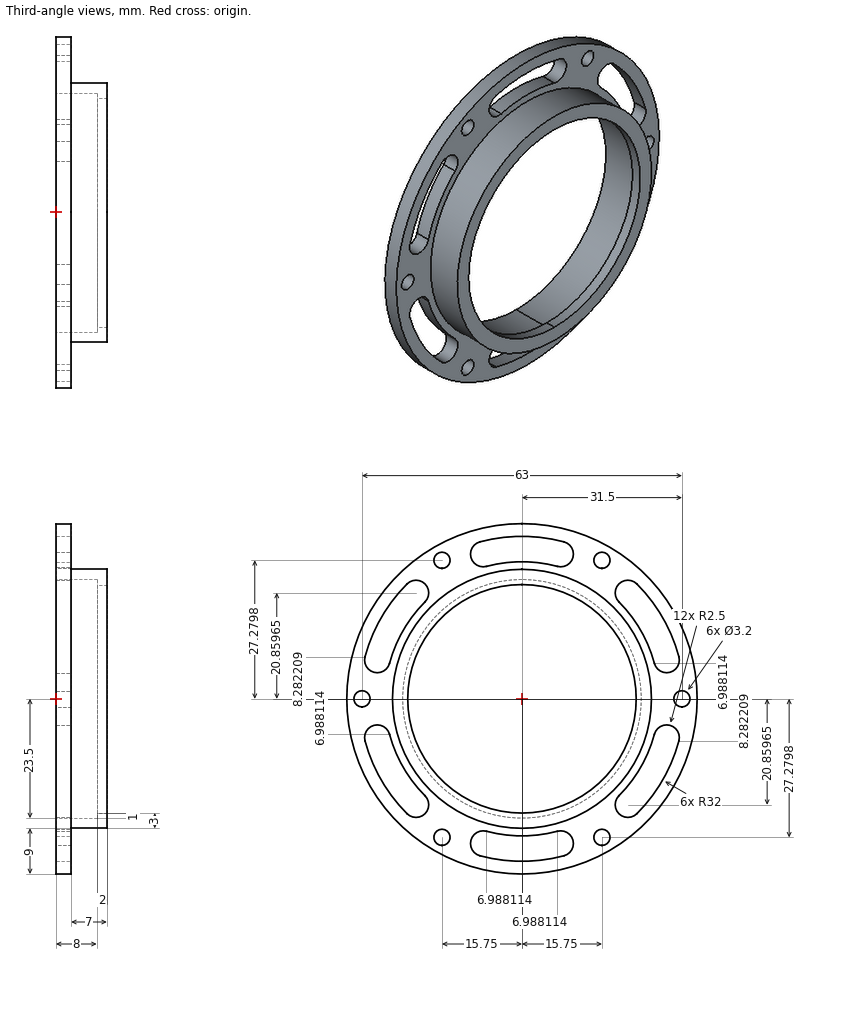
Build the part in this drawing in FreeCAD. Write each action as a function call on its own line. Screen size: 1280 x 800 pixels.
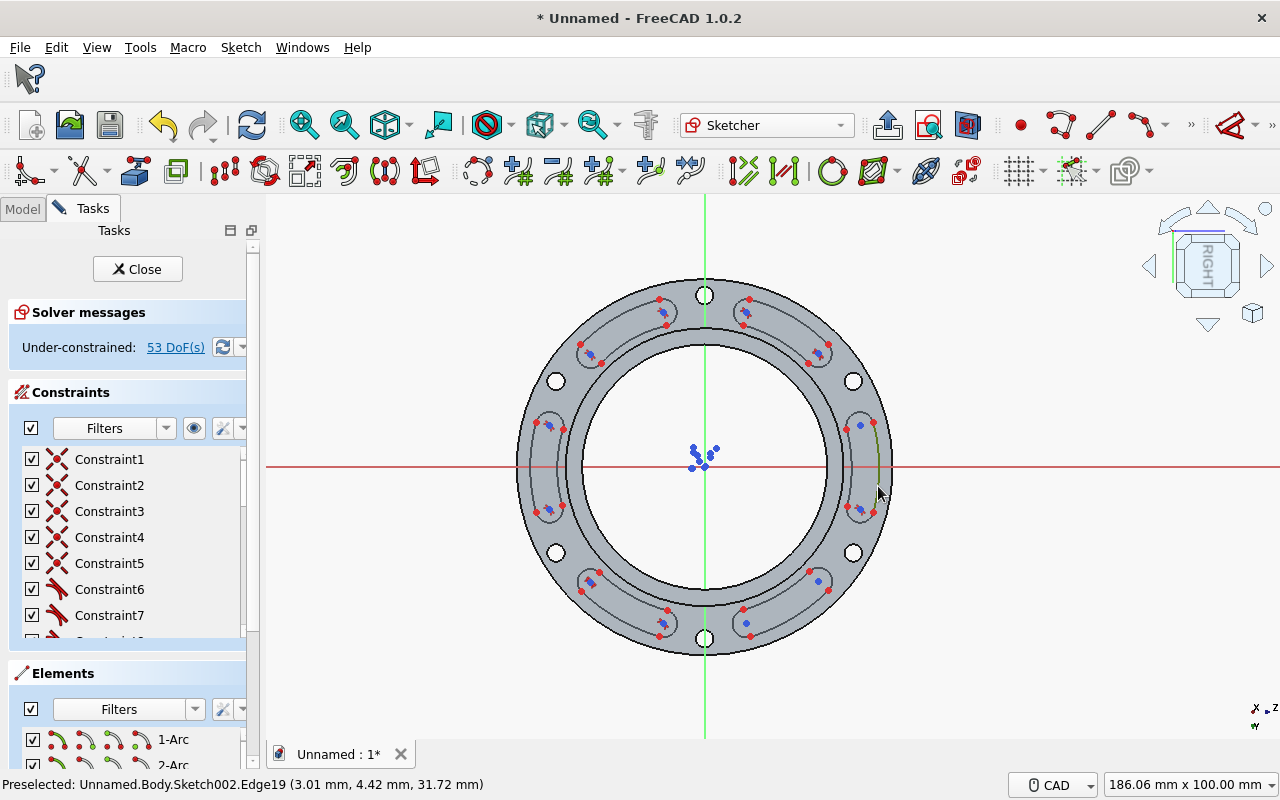
click(865, 413)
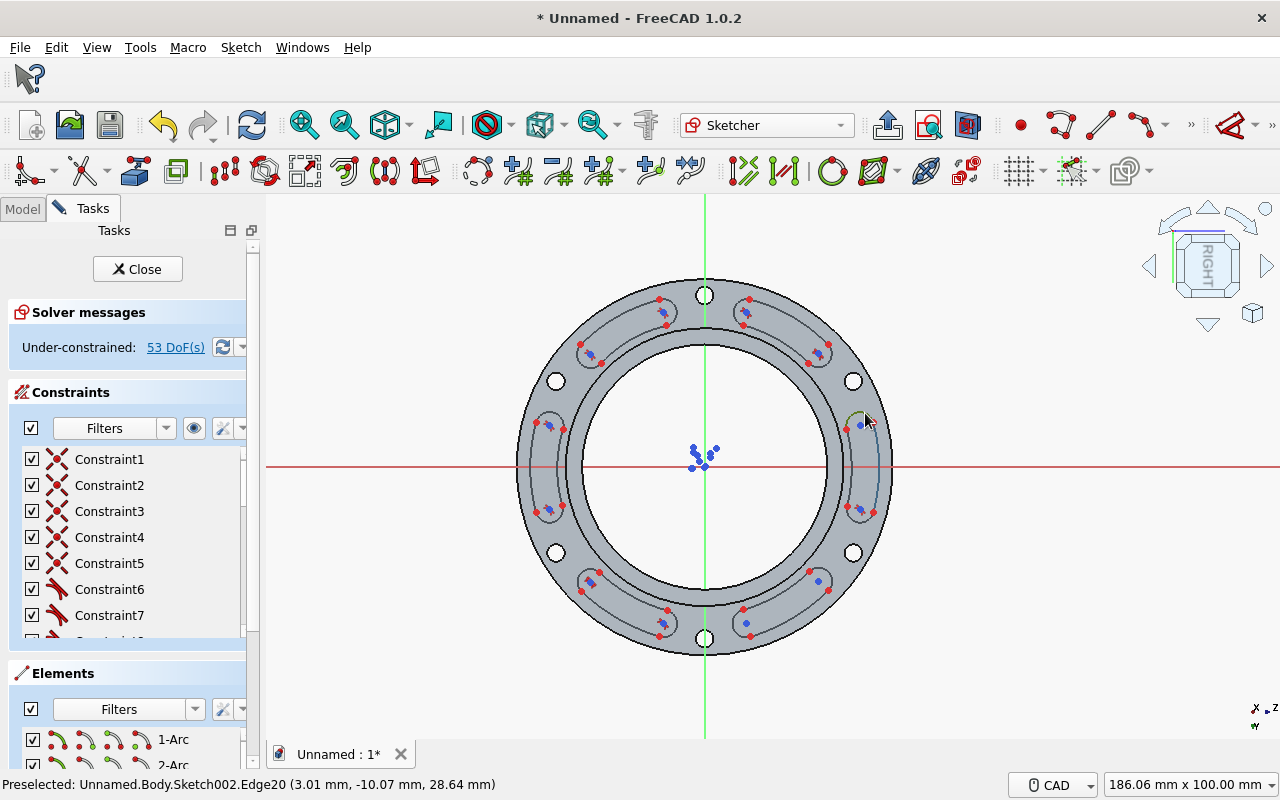
key(t)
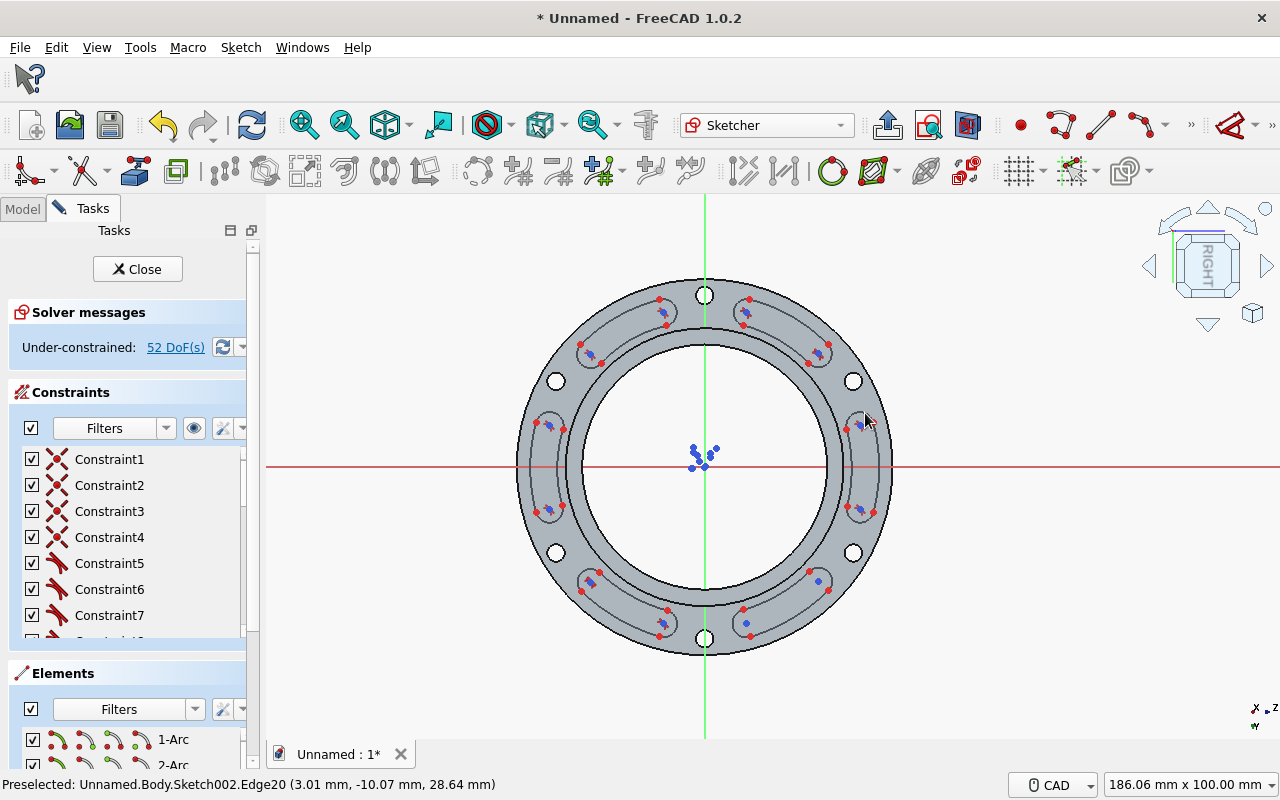
click(765, 602)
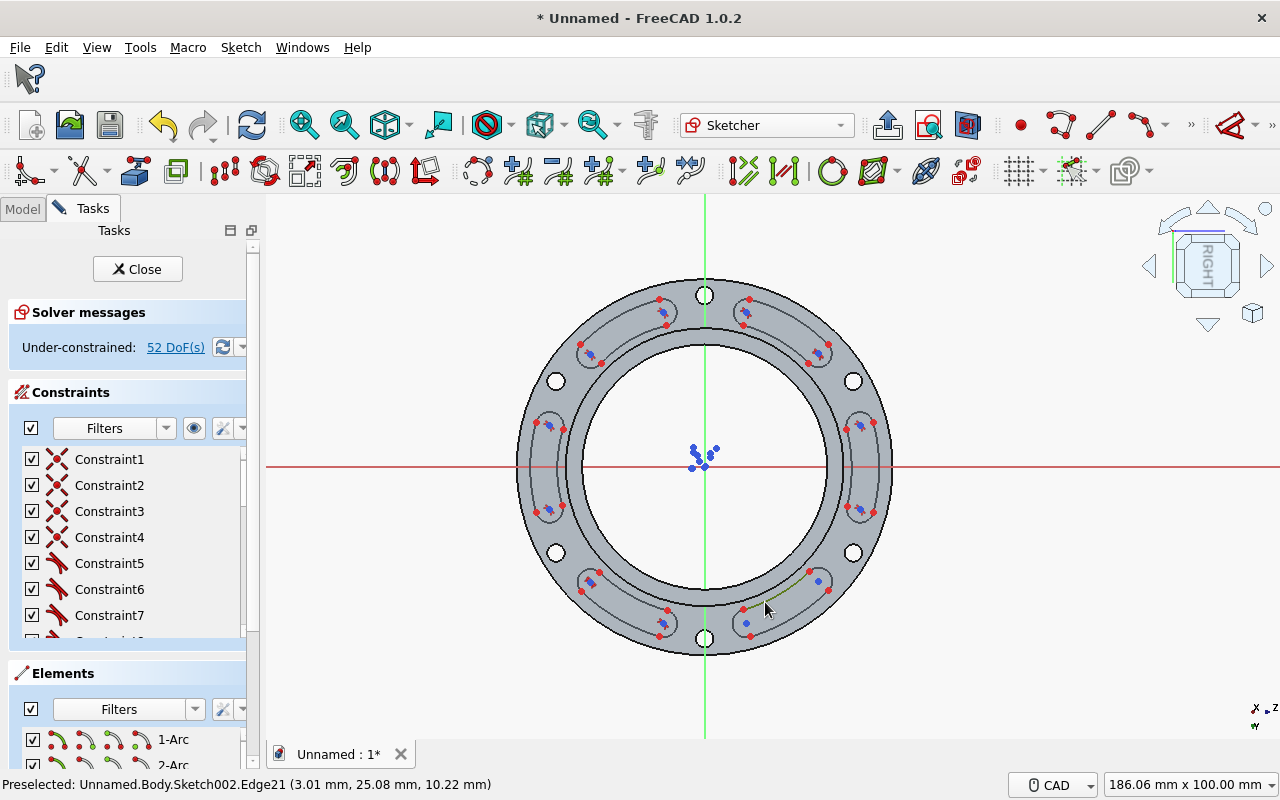
click(734, 618)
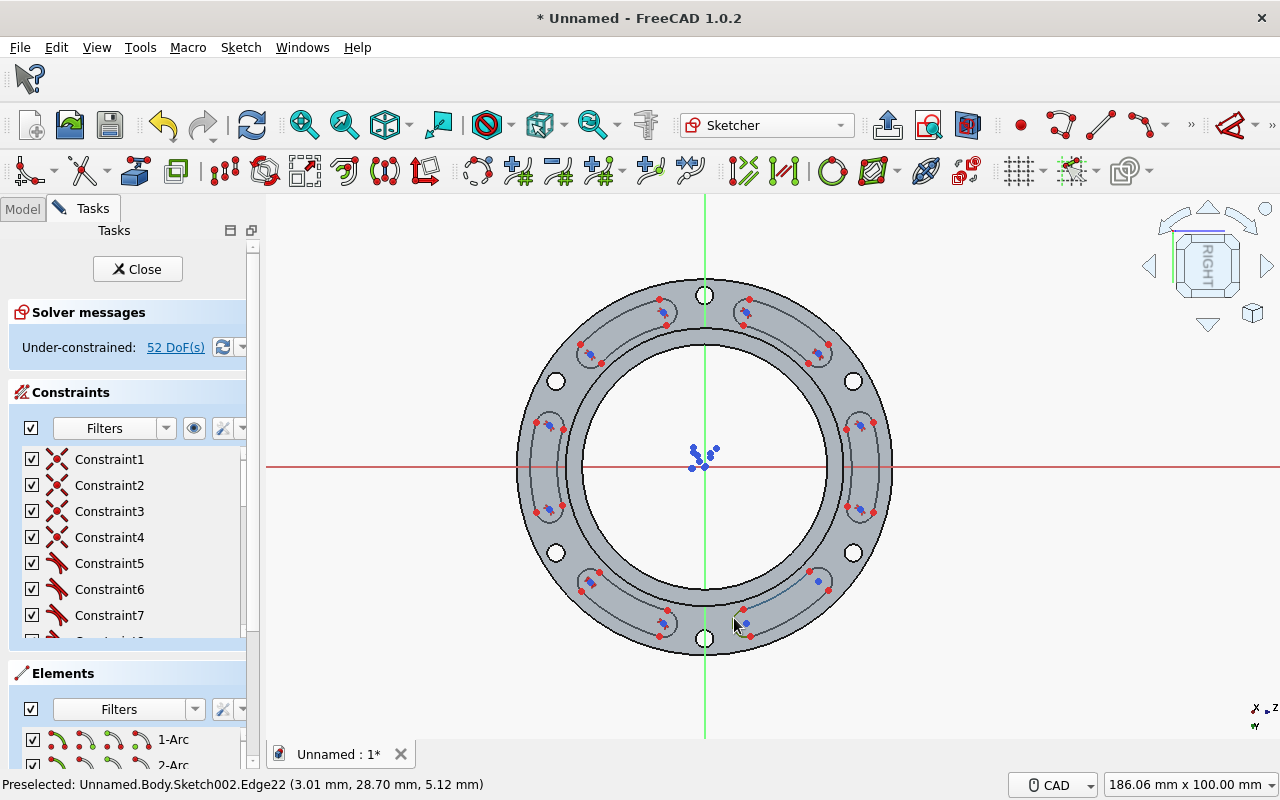
key(t)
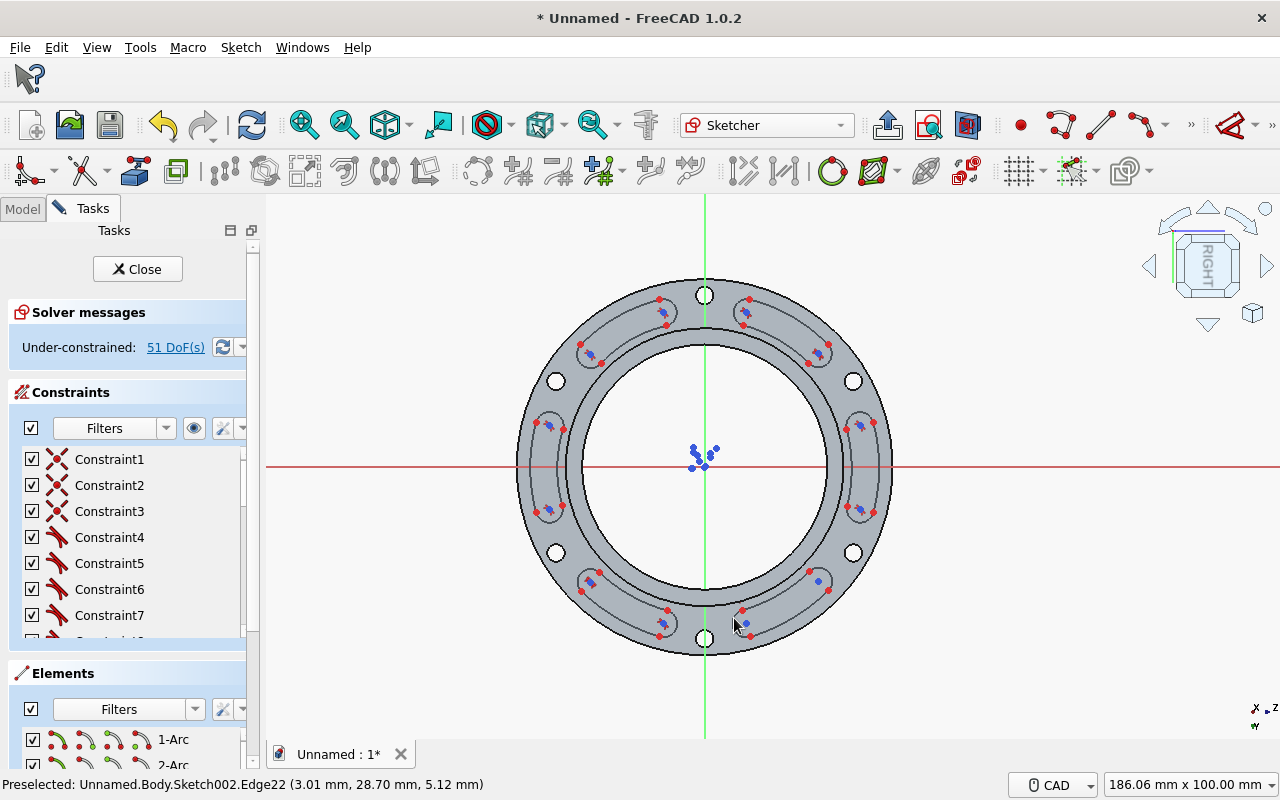
click(764, 602)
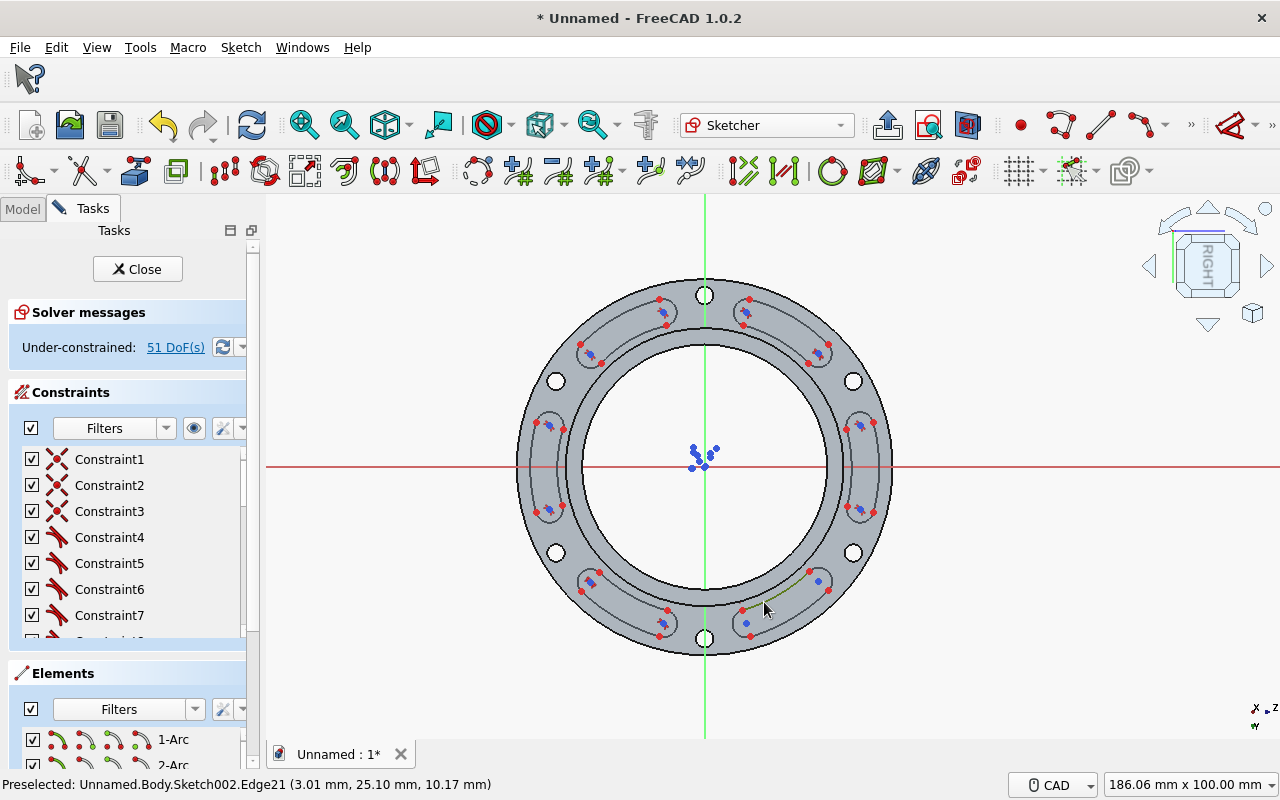
click(832, 579)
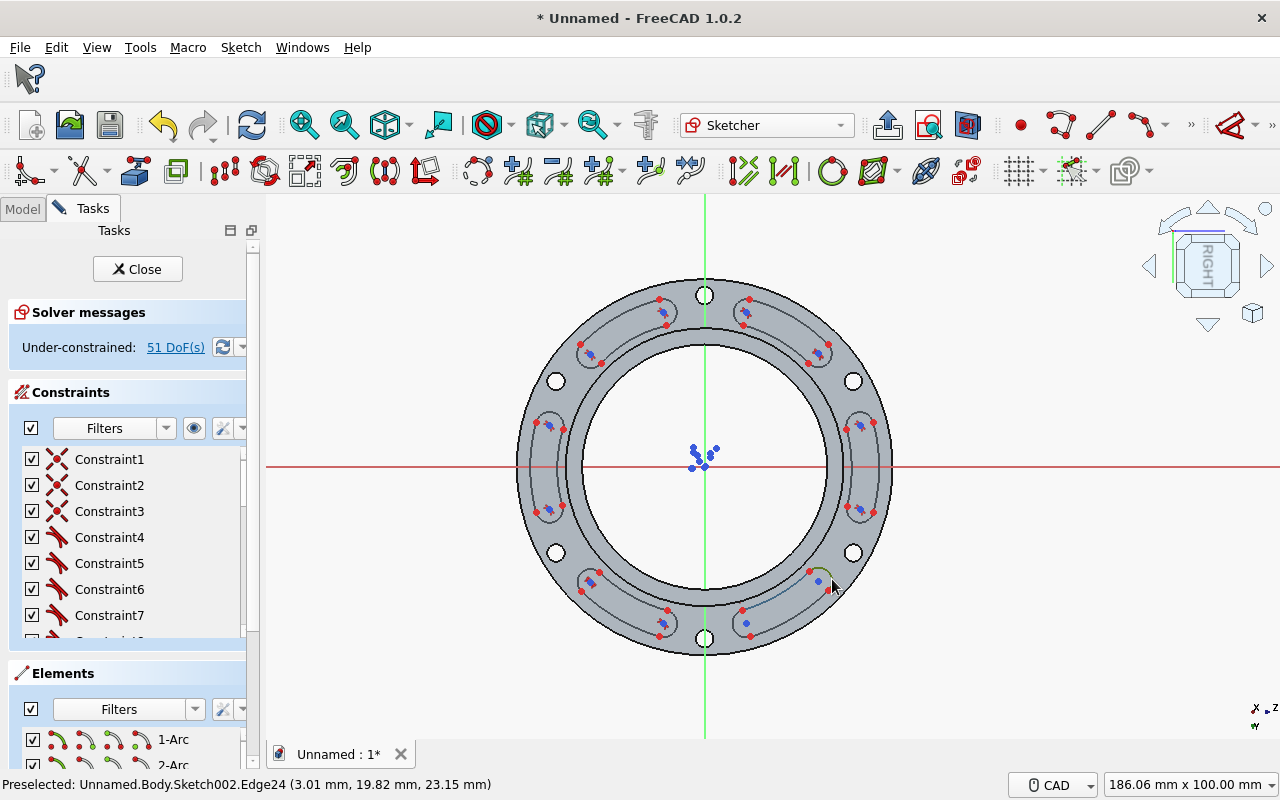
key(t)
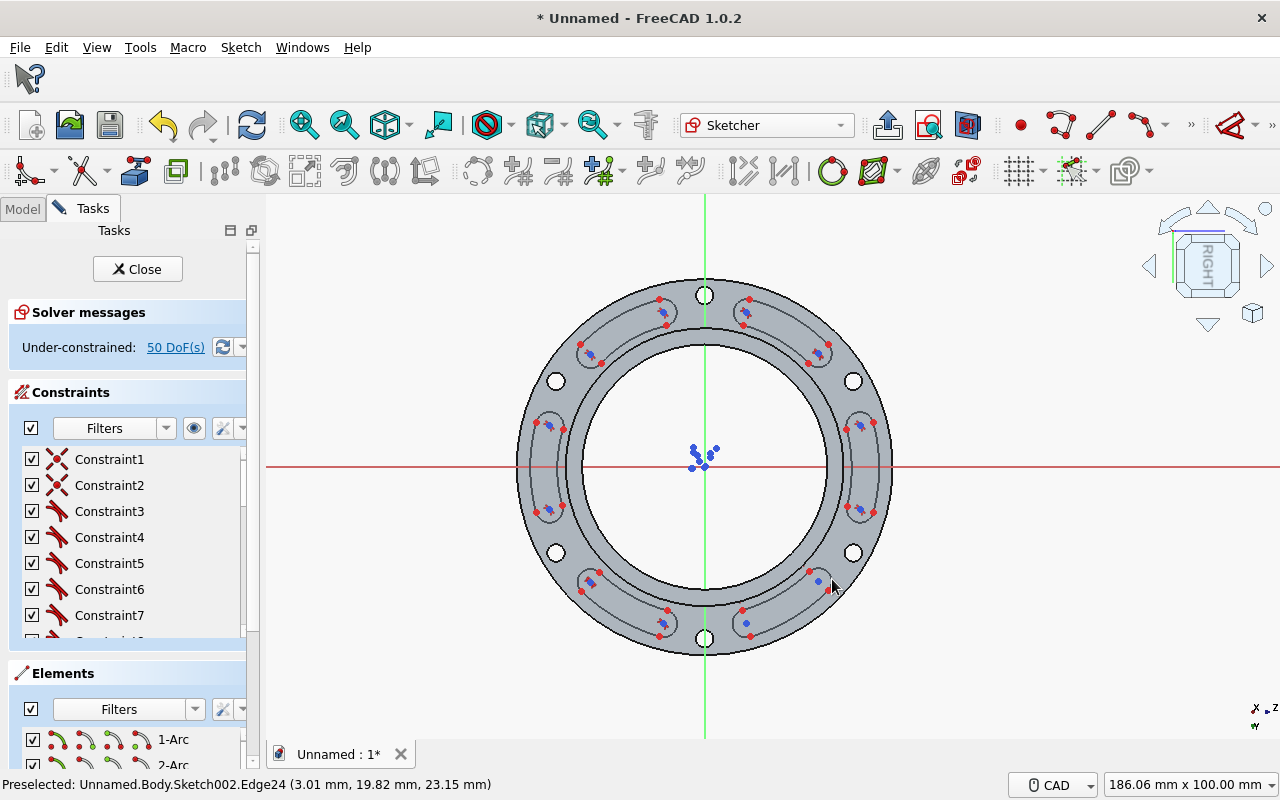
click(733, 619)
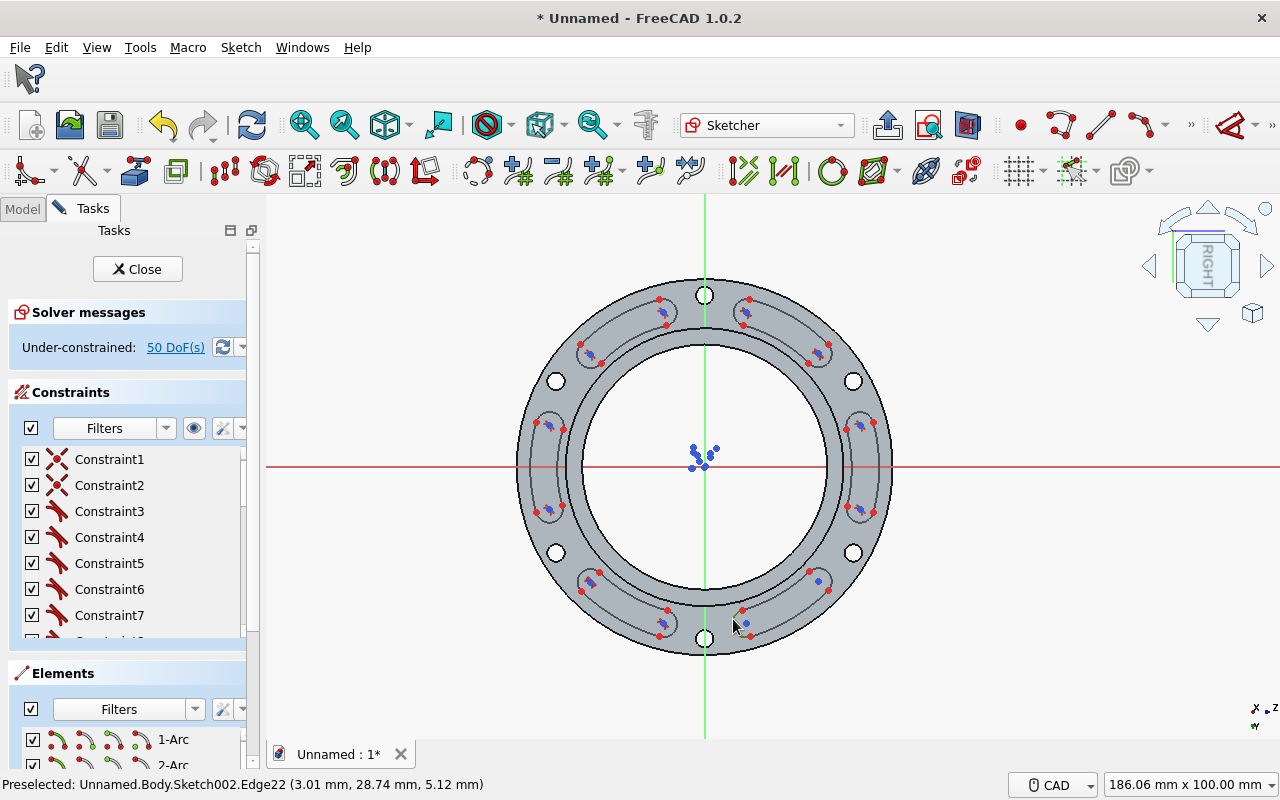
click(776, 627)